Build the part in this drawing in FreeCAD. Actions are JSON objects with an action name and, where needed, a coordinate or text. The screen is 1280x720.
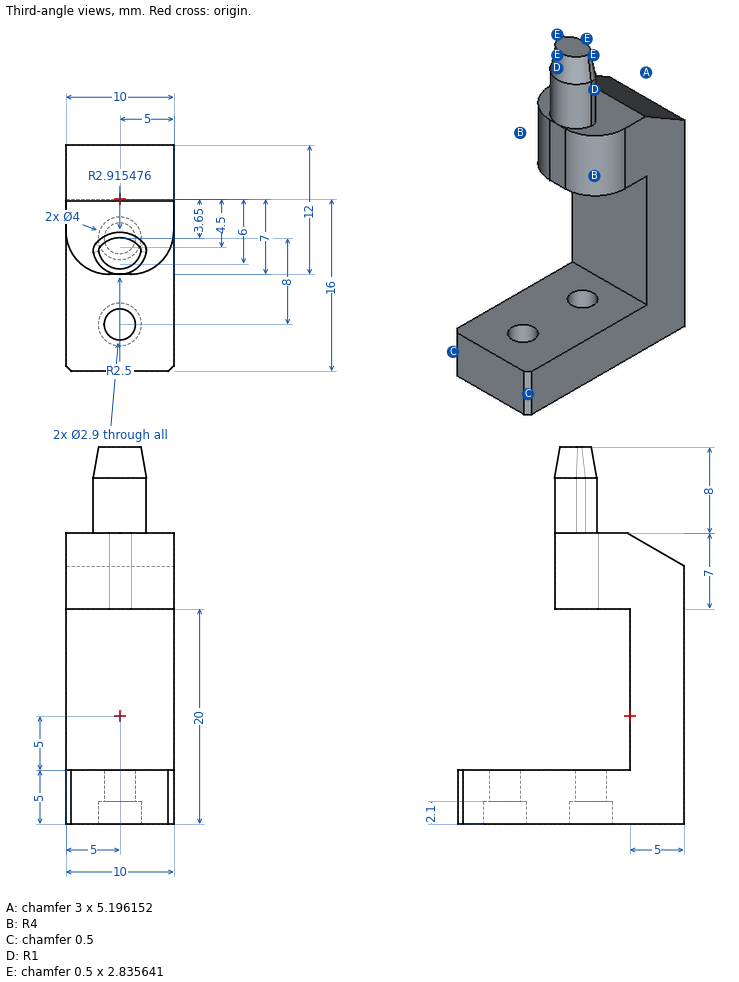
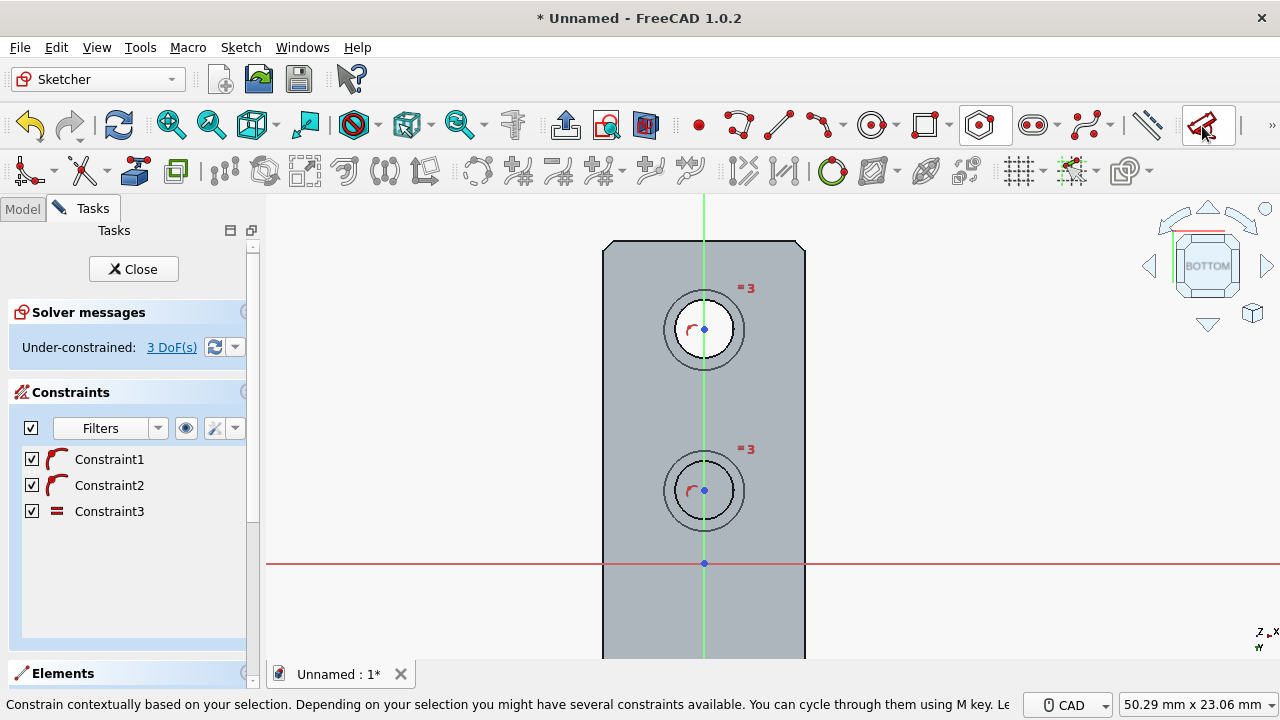
{"action": "left_click", "coordinate": [733, 463]}
{"action": "left_click", "coordinate": [756, 441]}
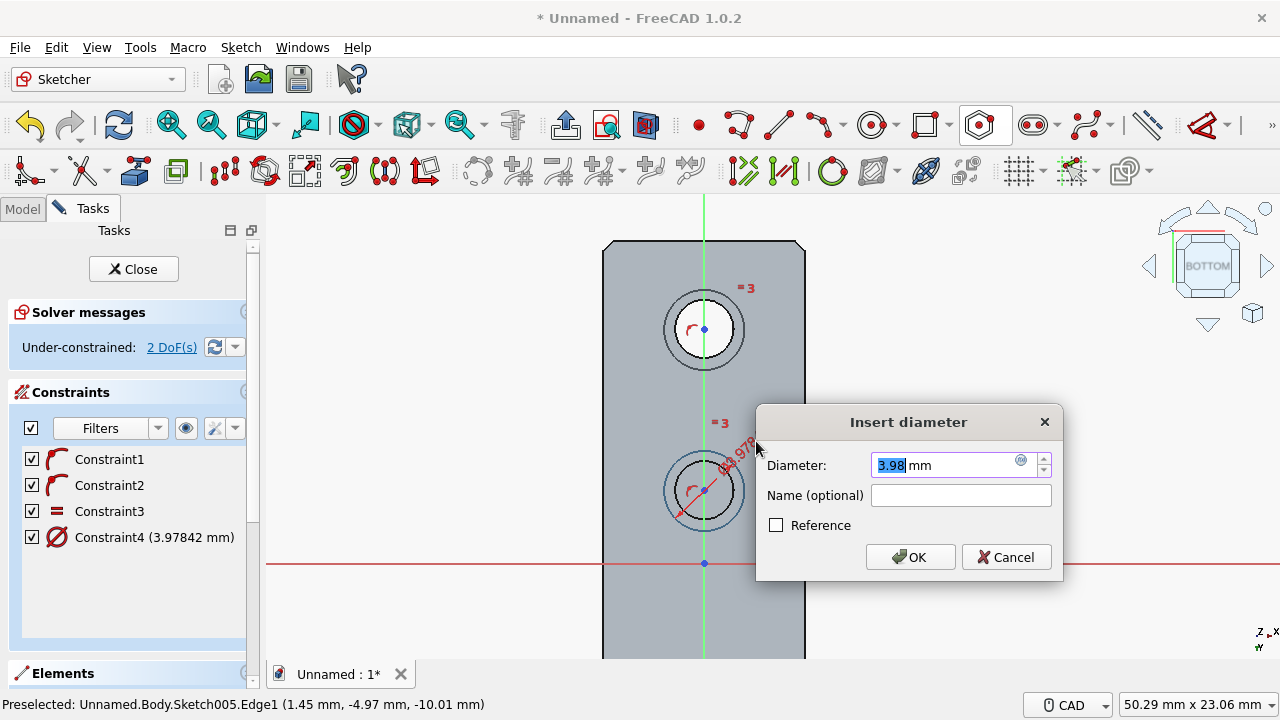
{"action": "type", "text": "4"}
{"action": "key", "text": "Return"}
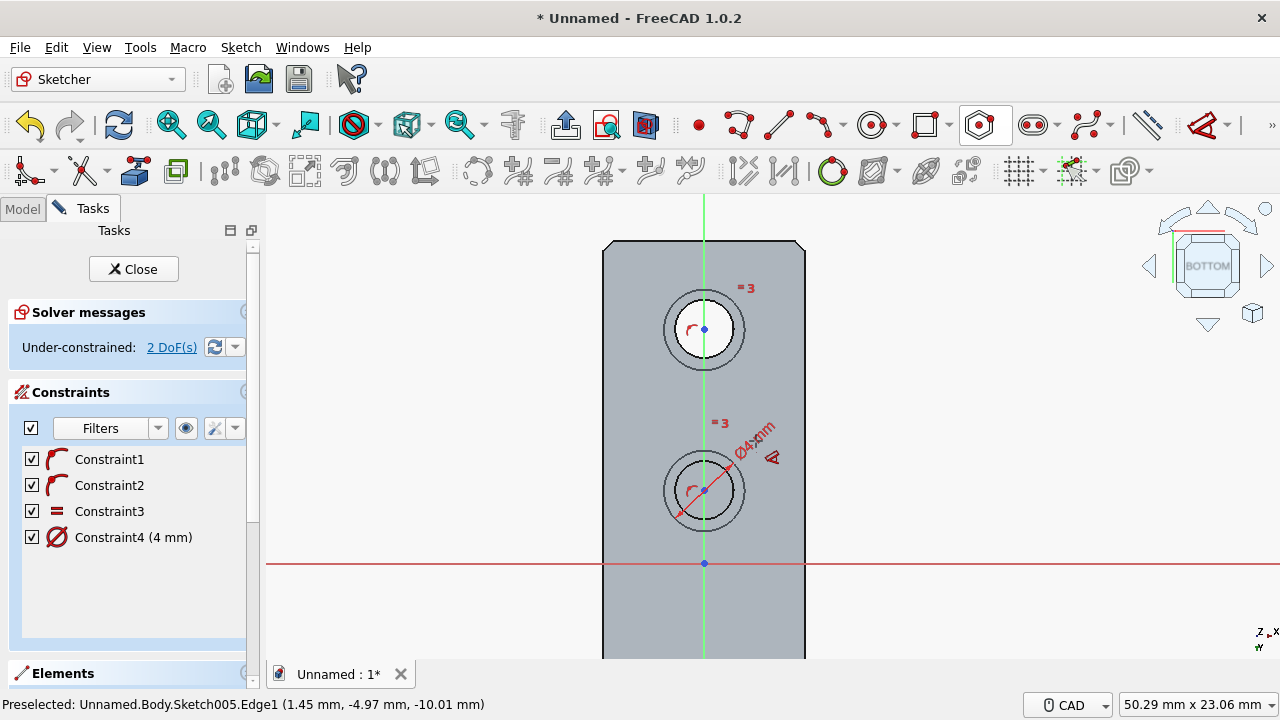
{"action": "left_click", "coordinate": [704, 491]}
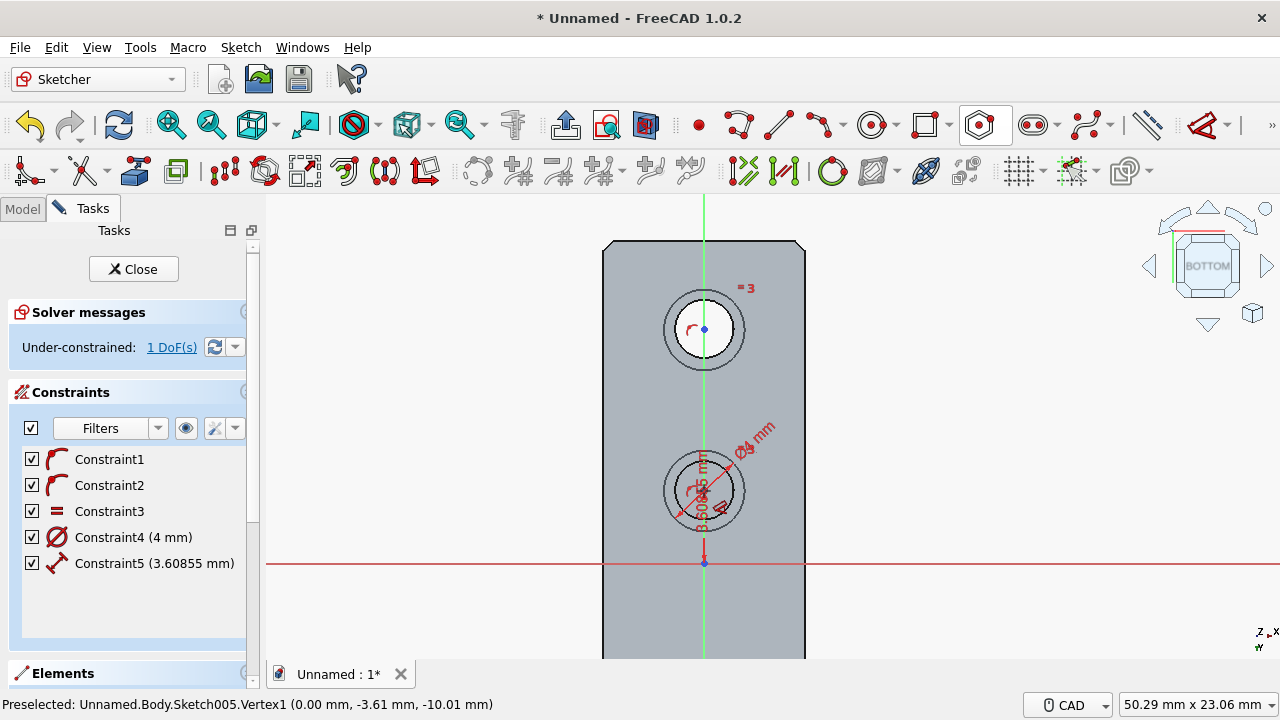
{"action": "left_click", "coordinate": [704, 330]}
{"action": "left_click", "coordinate": [738, 410]}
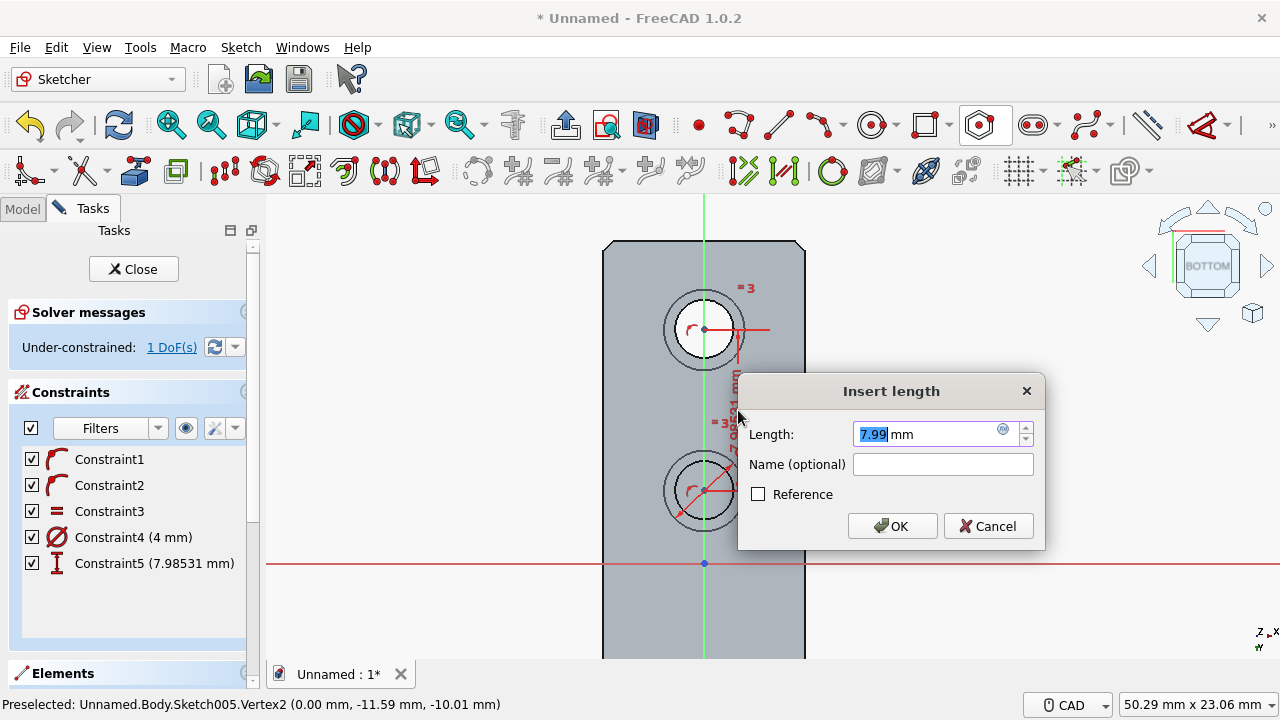
{"action": "type", "text": "8"}
{"action": "key", "text": "Return"}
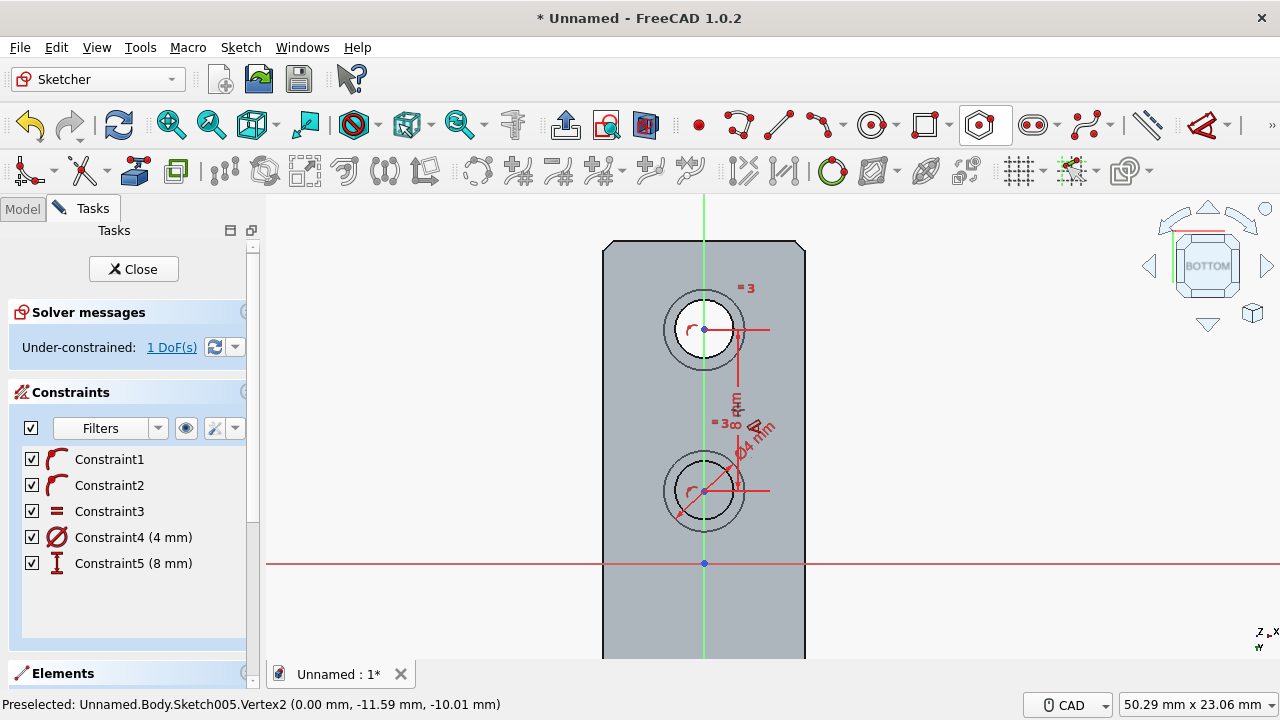
{"action": "left_click", "coordinate": [704, 491]}
{"action": "left_click", "coordinate": [738, 544]}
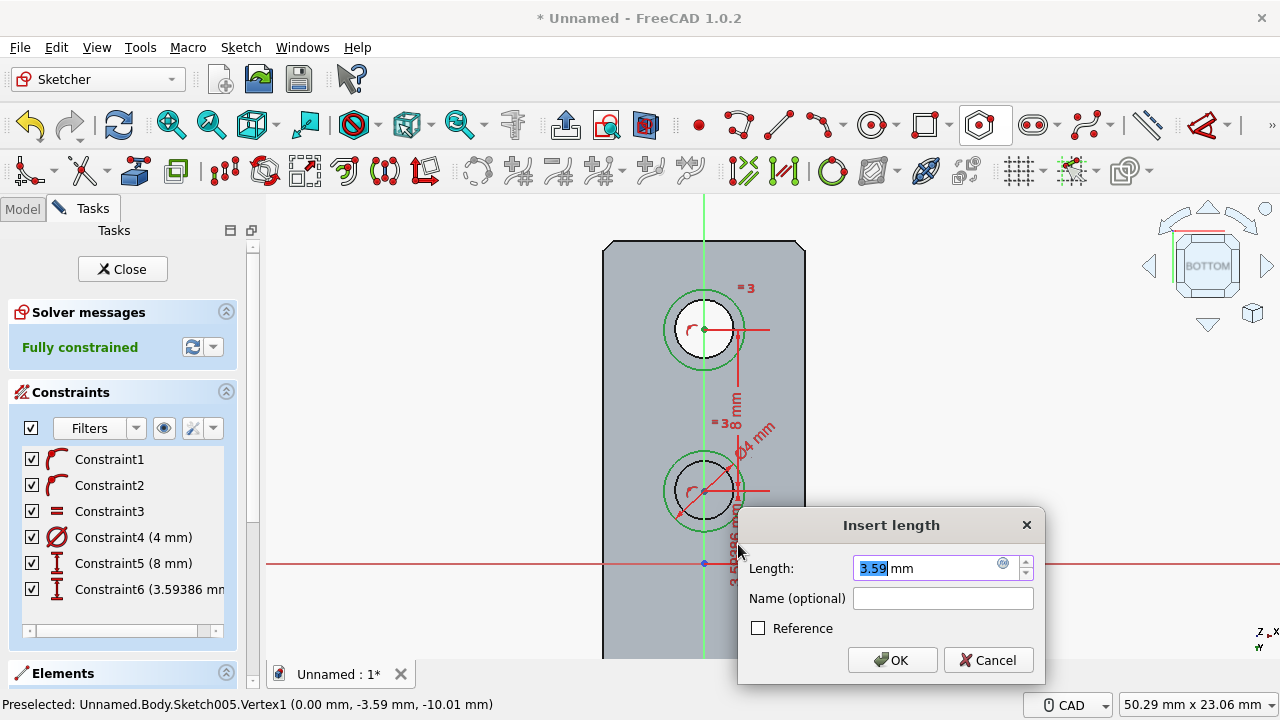
{"action": "type", "text": "3.65"}
{"action": "key", "text": "Return"}
{"action": "key", "text": "Escape"}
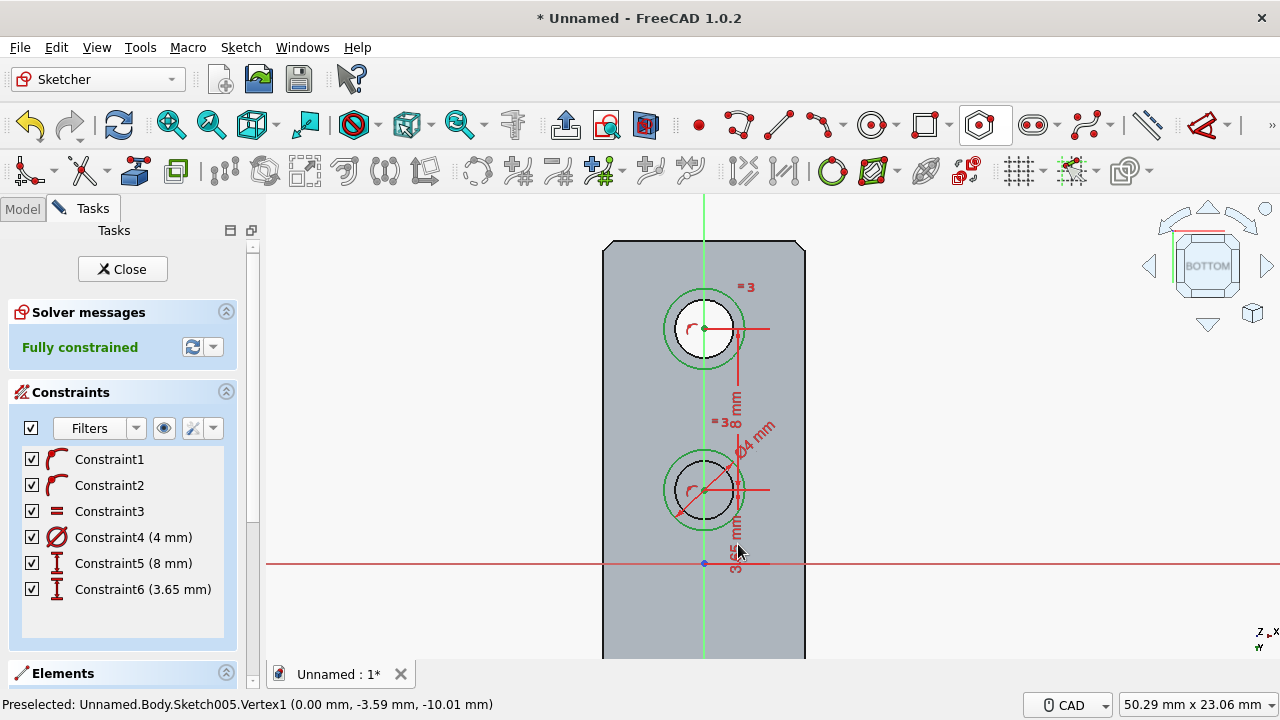
{"action": "left_click", "coordinate": [123, 269]}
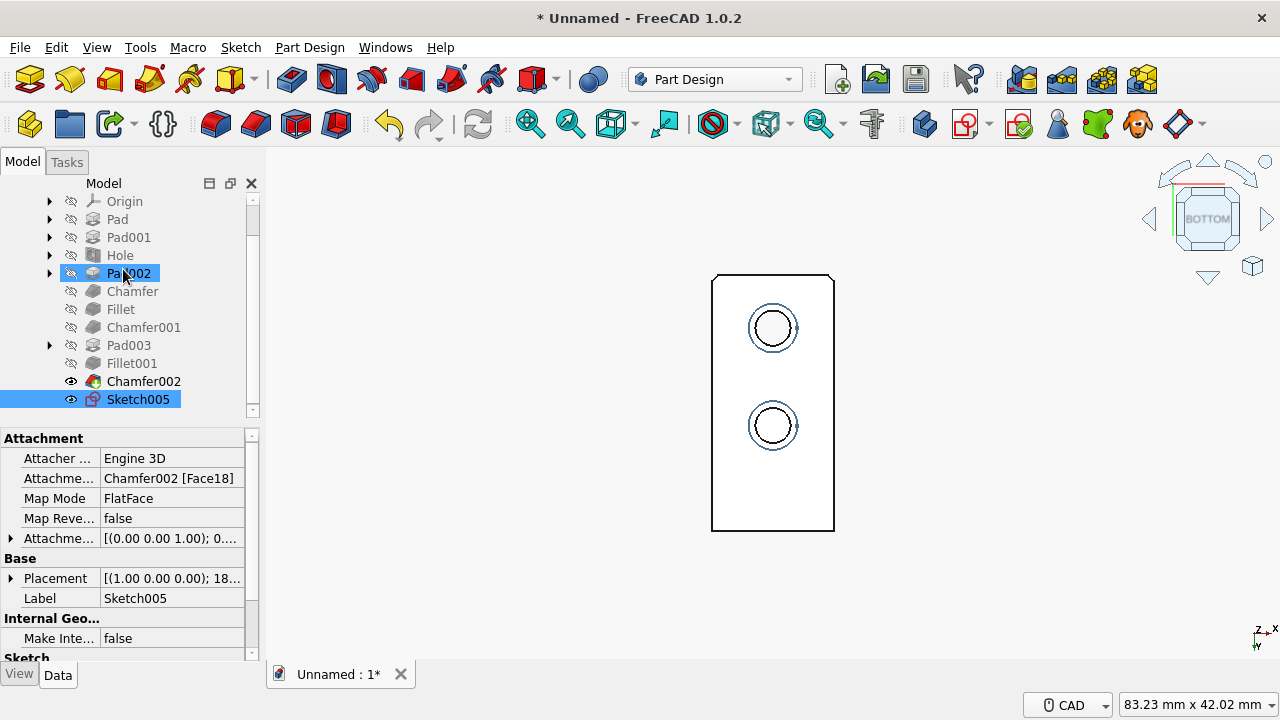
{"action": "left_click", "coordinate": [292, 80]}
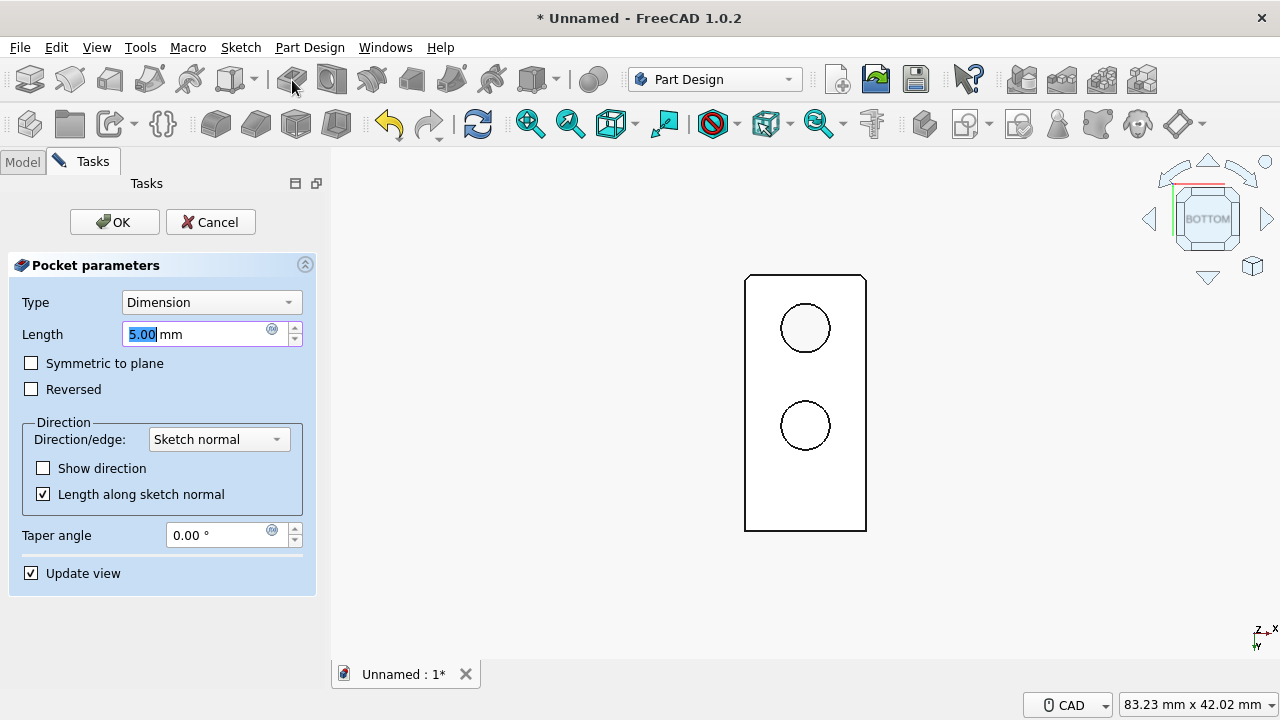
{"action": "type", "text": "2.1"}
{"action": "key", "text": "Tab"}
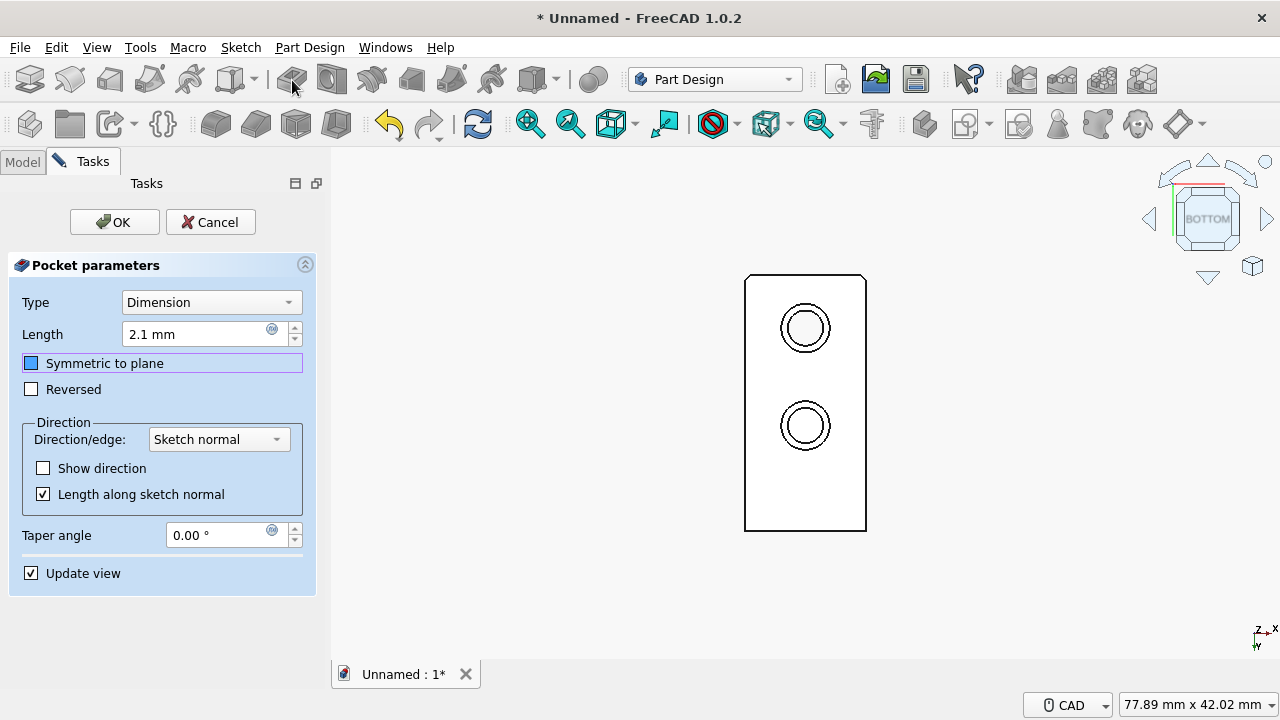
{"action": "left_click", "coordinate": [115, 222]}